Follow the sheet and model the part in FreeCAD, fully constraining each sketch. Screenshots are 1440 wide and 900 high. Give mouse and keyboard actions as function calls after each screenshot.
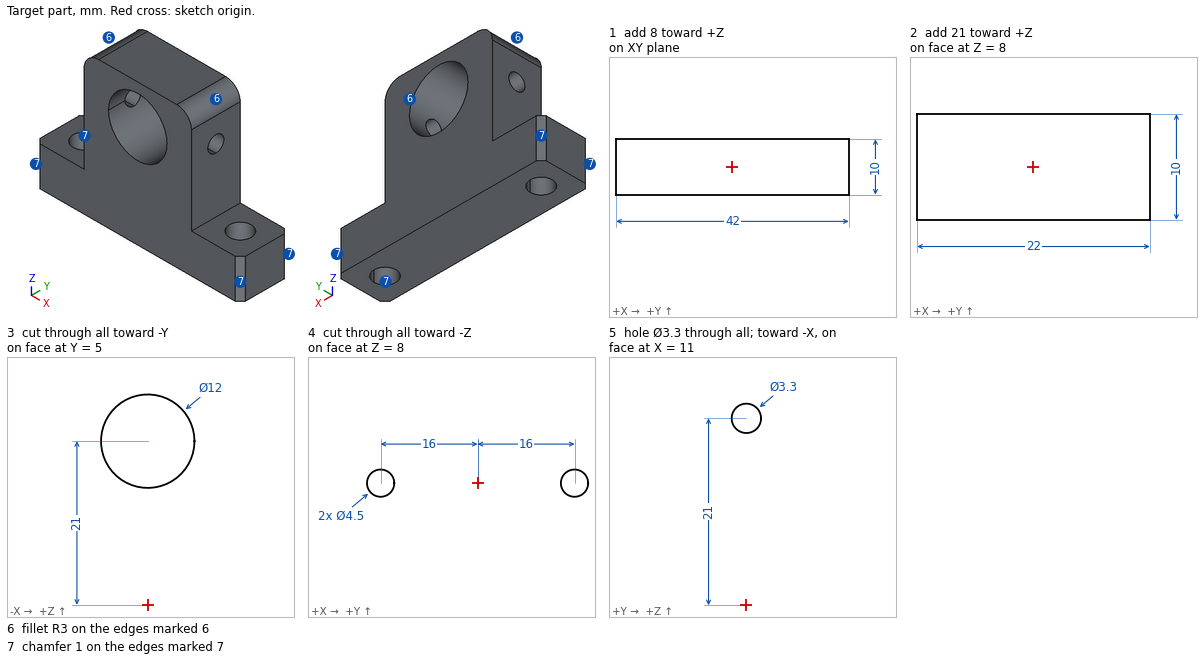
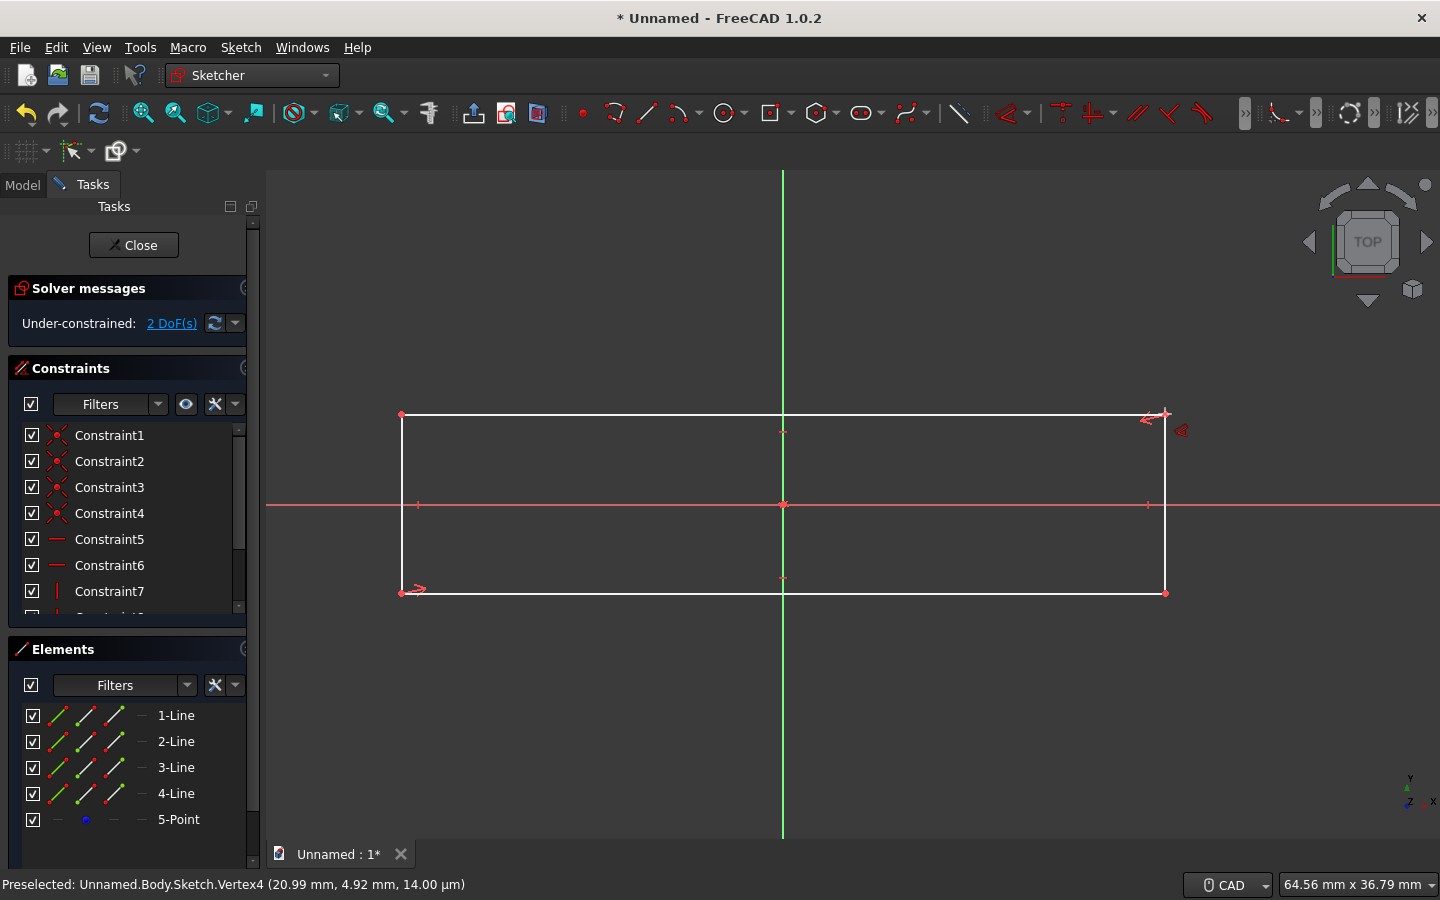
click(631, 594)
click(608, 628)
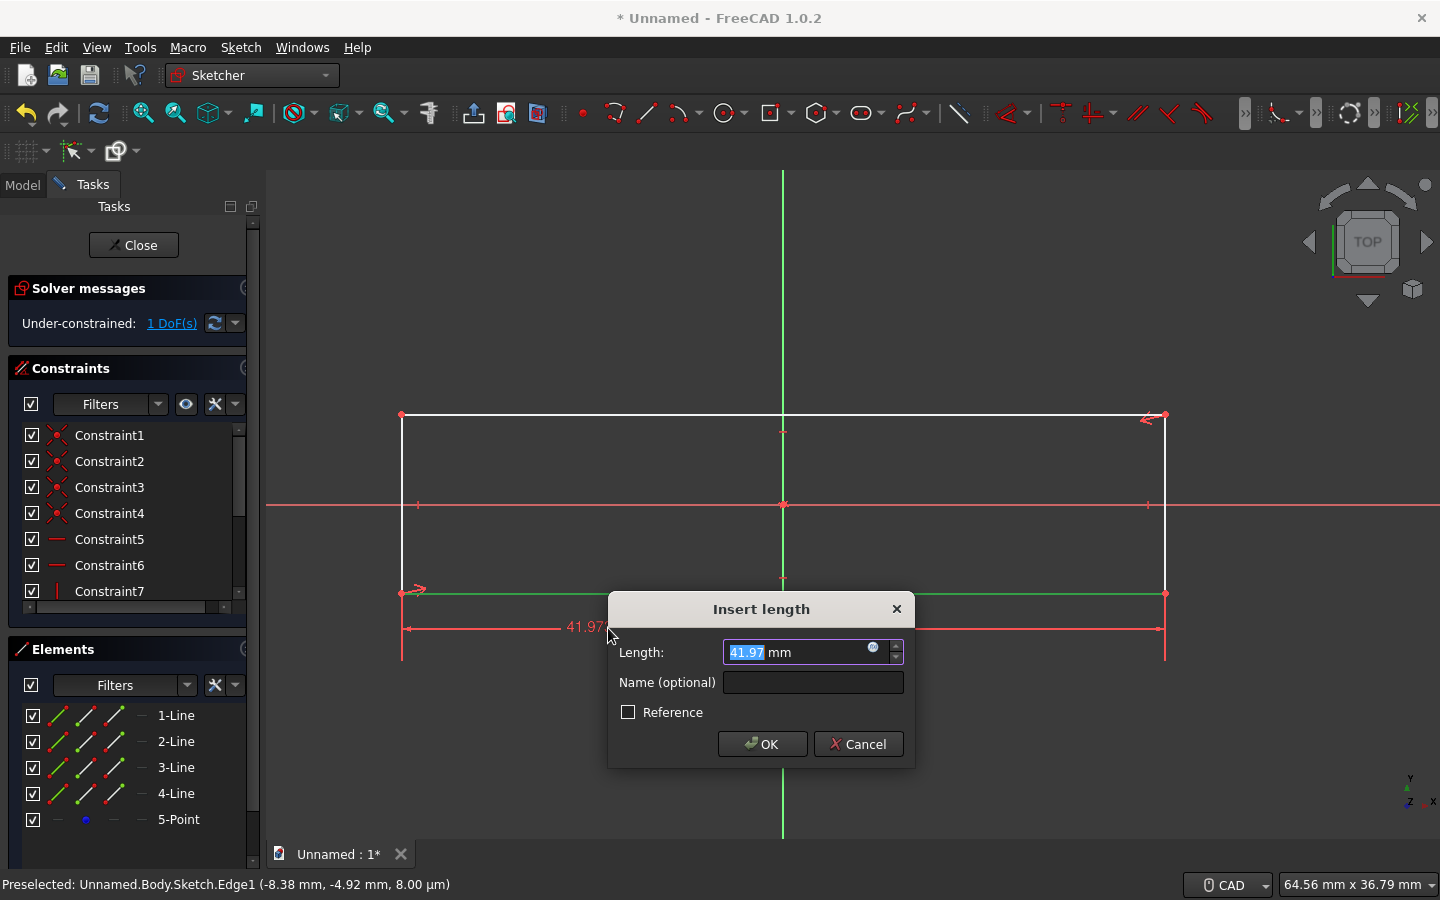
text(42)
key(Return)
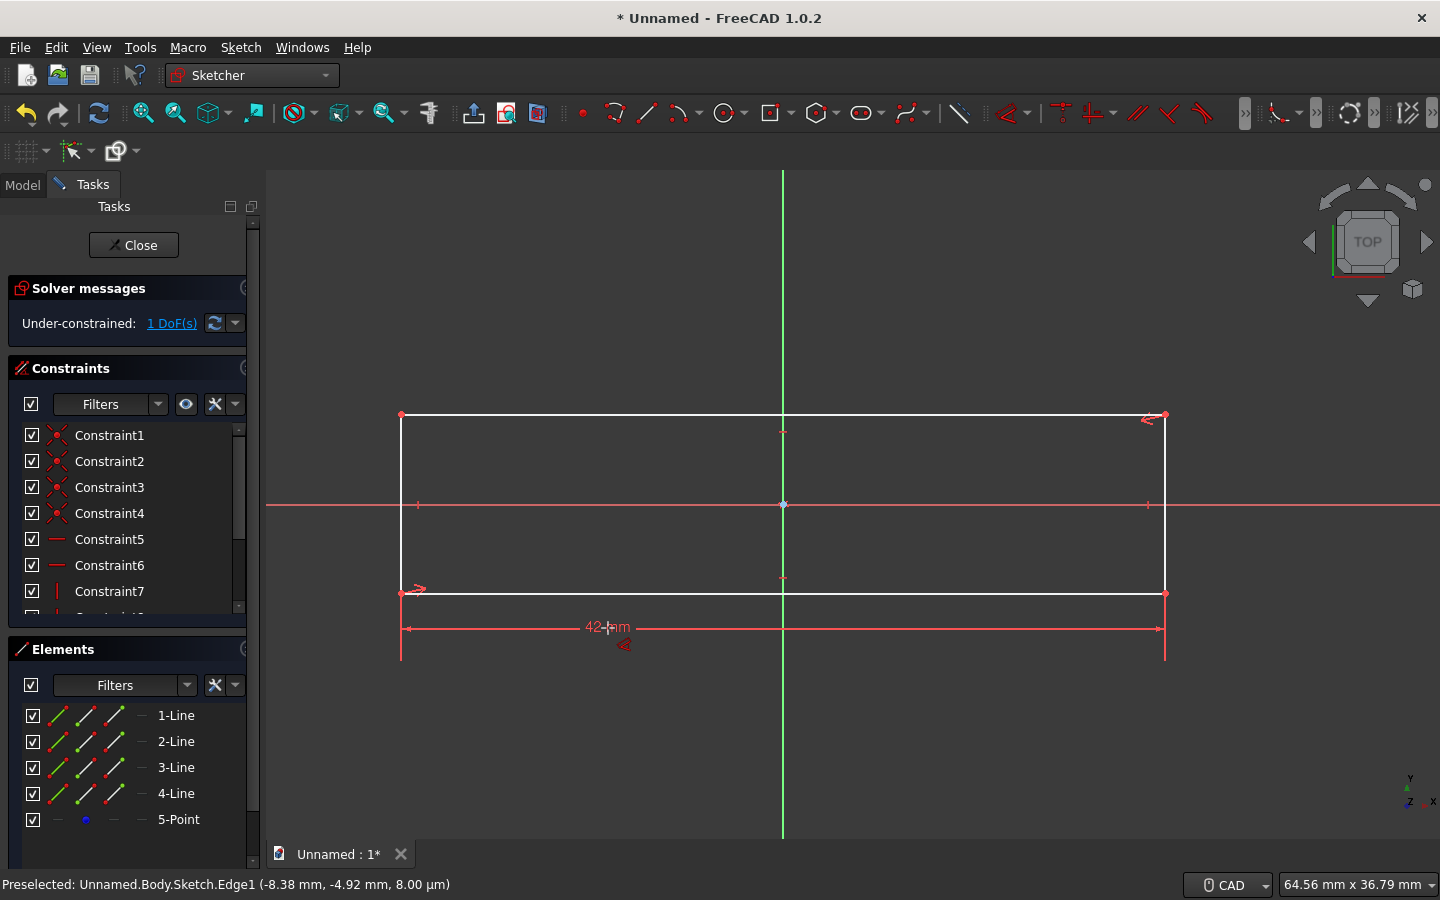
click(1165, 540)
click(1199, 463)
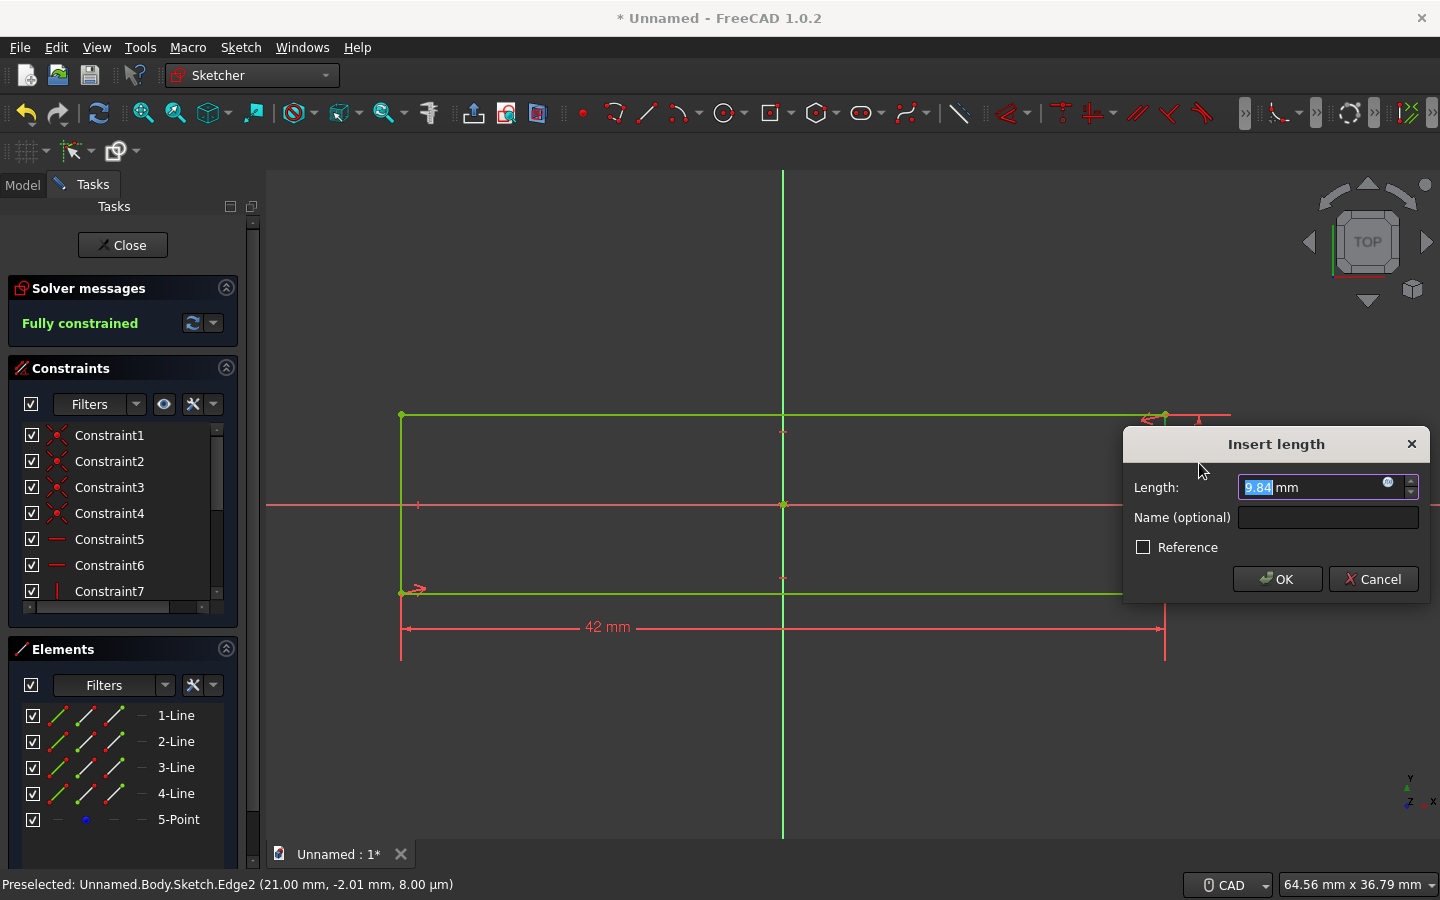
text(10)
key(Return)
key(Escape)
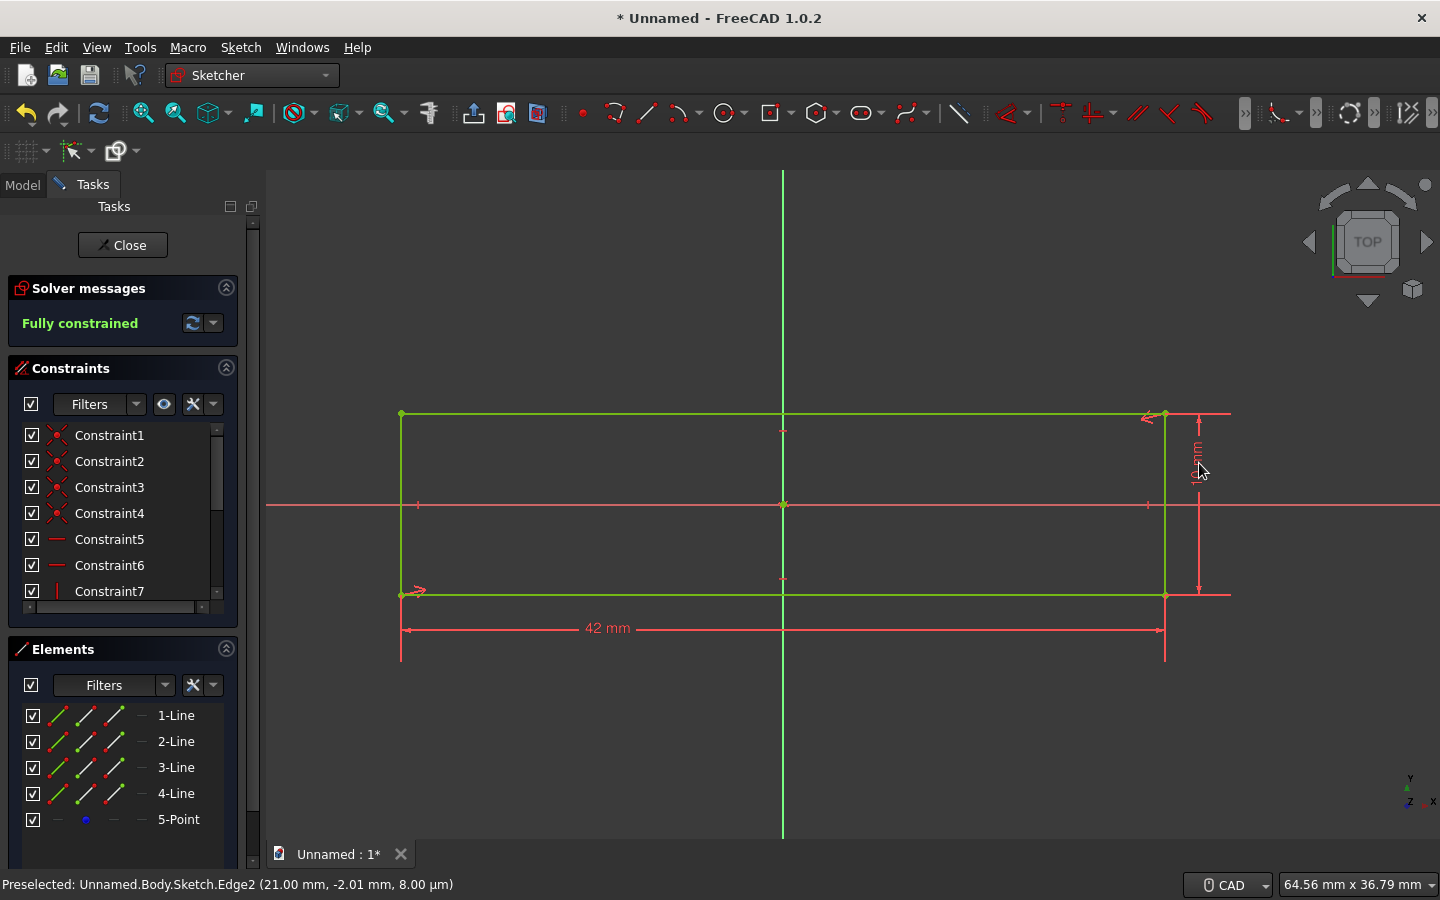
click(123, 245)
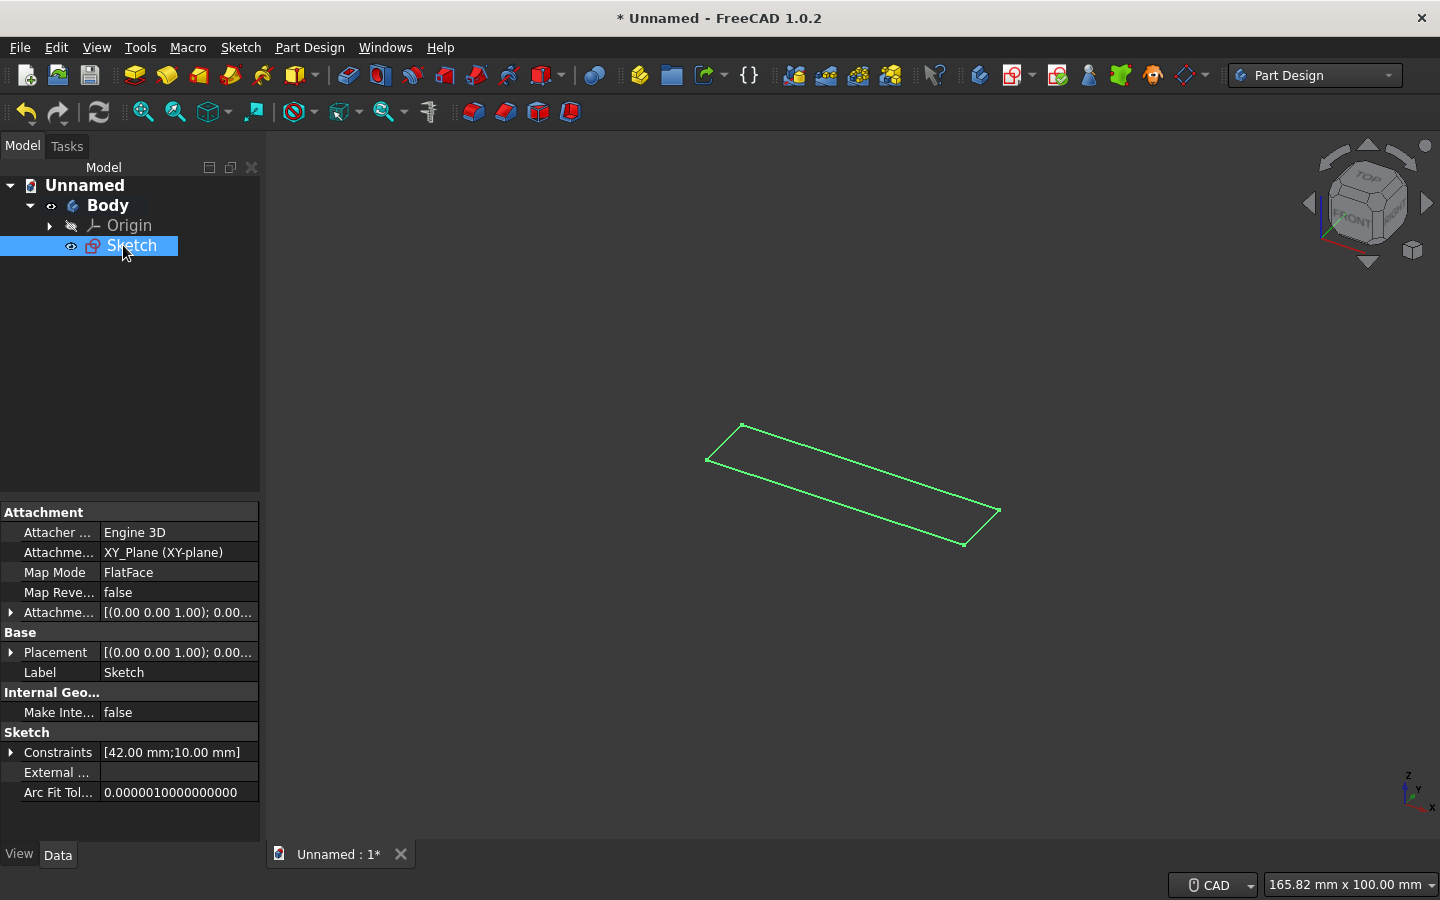
click(136, 76)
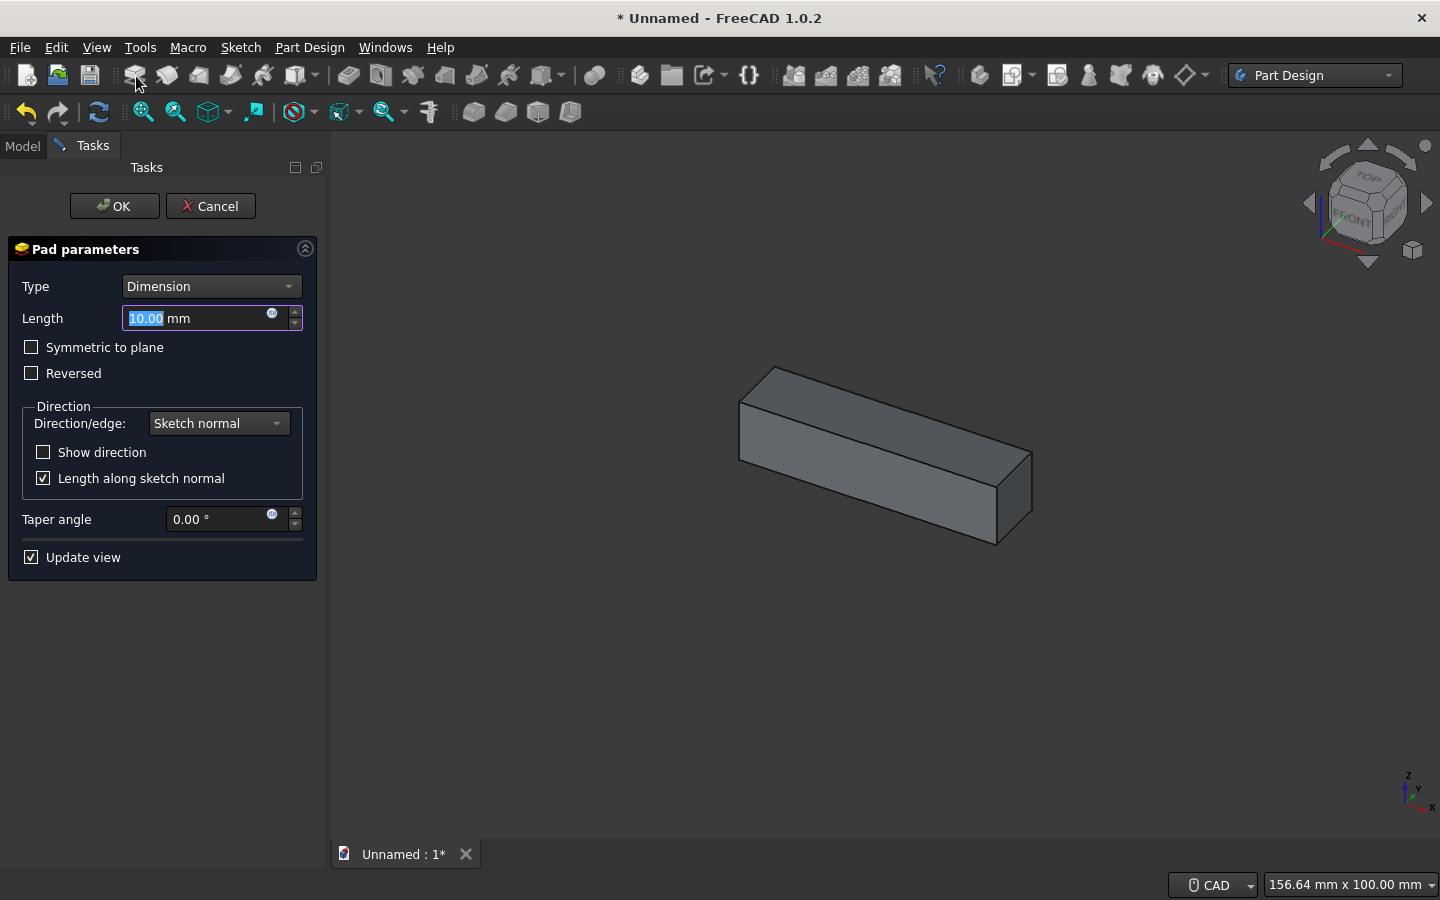
text(8)
key(Tab)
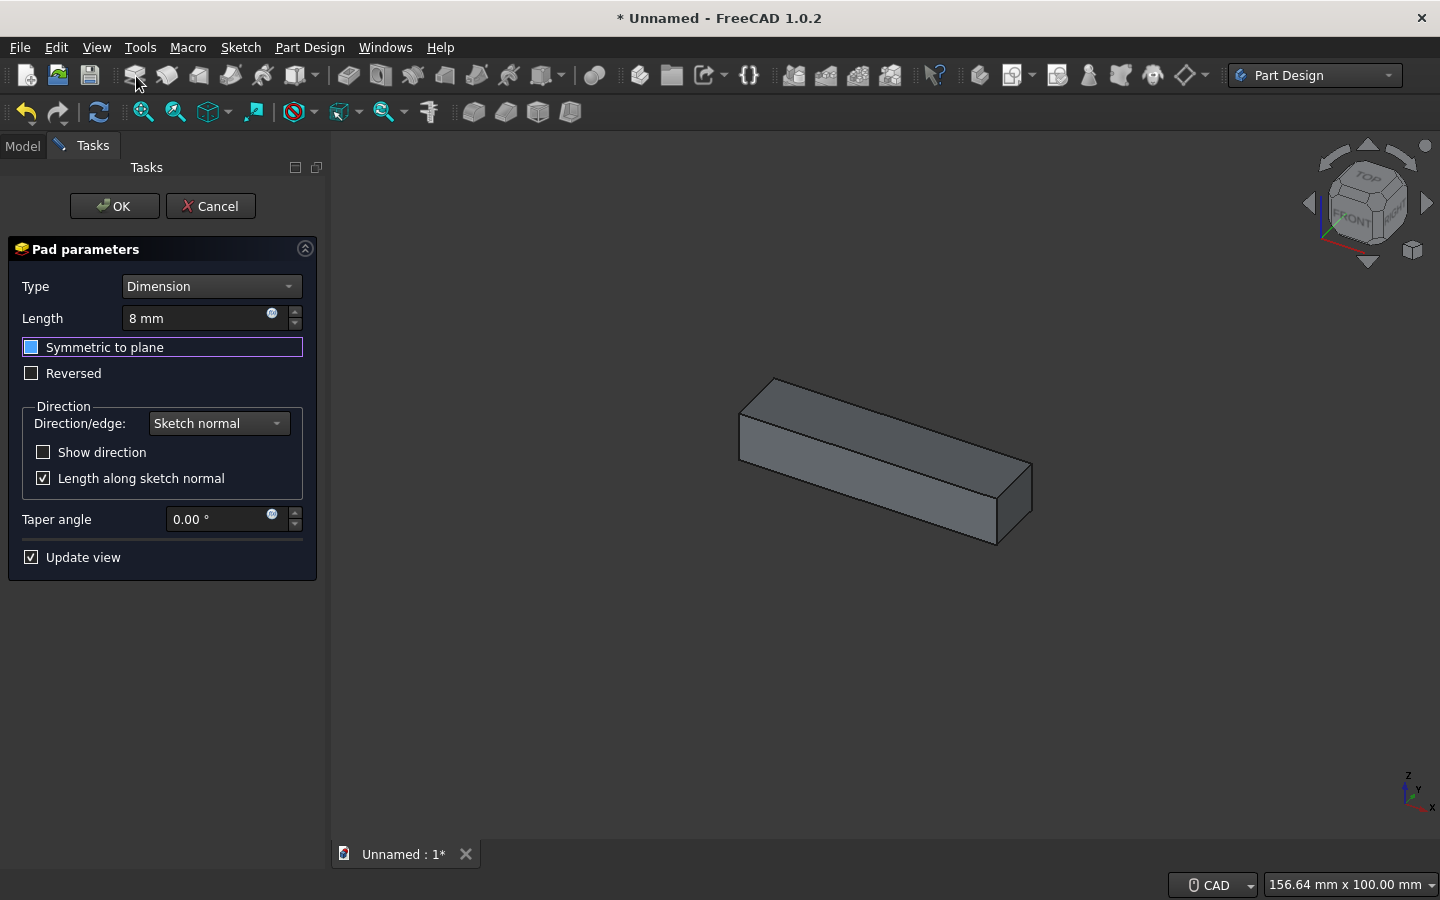
click(115, 206)